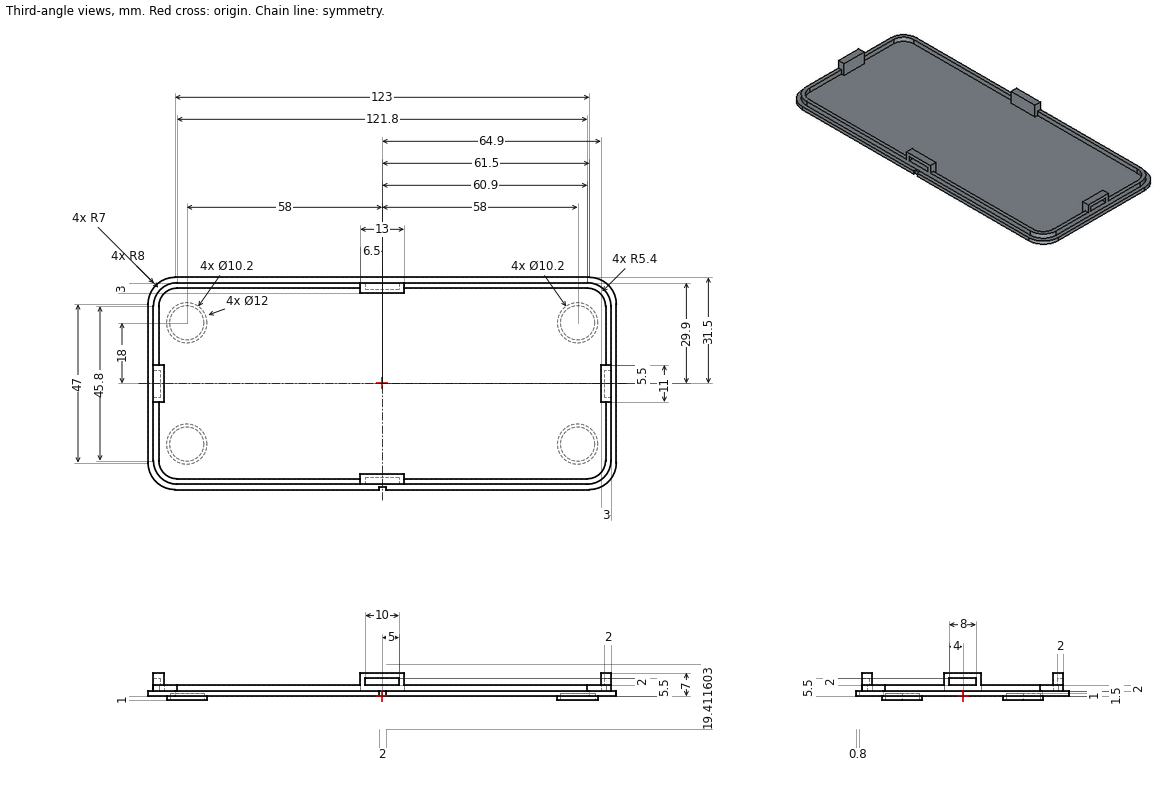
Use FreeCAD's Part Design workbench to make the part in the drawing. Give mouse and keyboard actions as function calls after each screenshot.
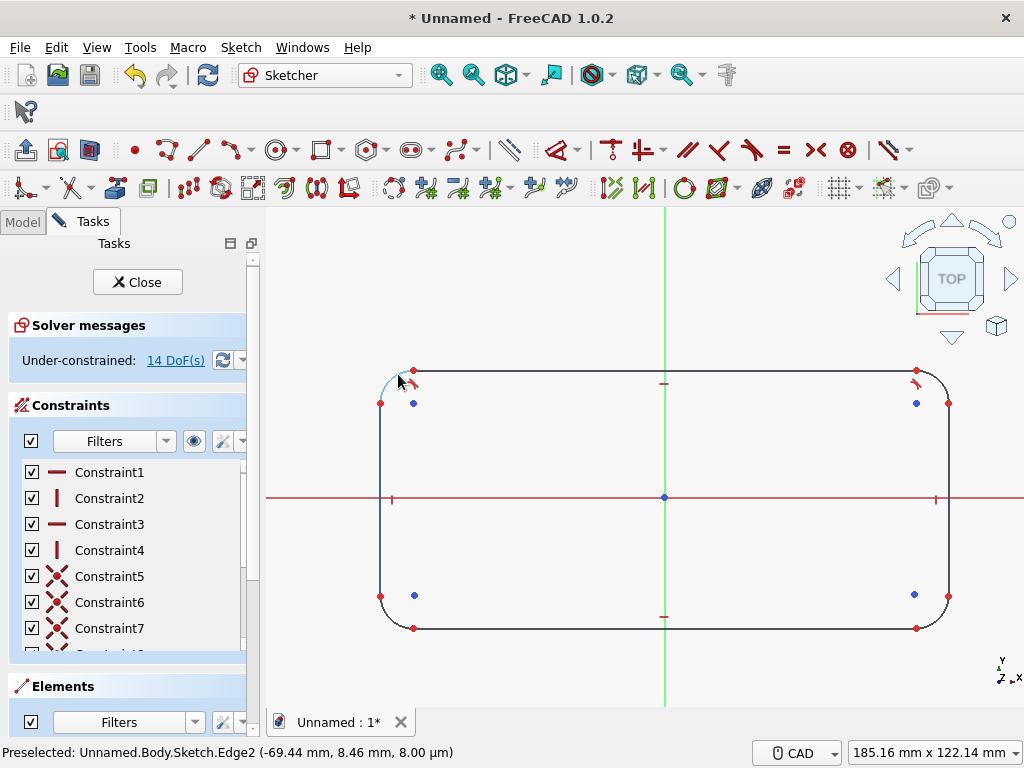
click(398, 374)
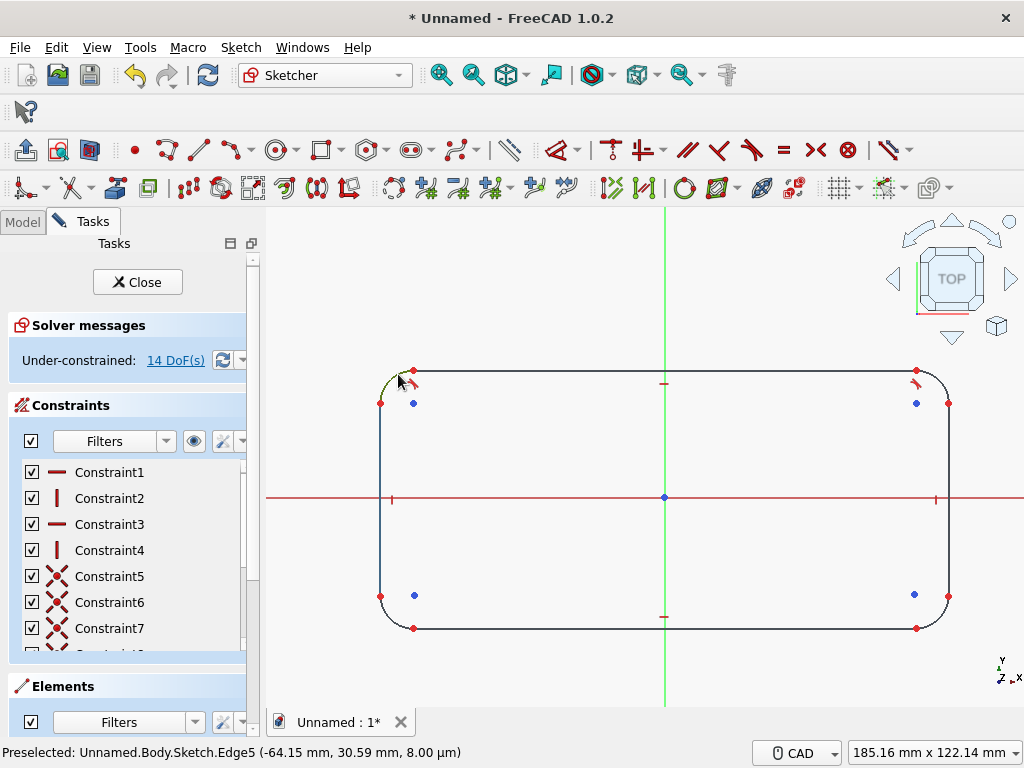
key(t)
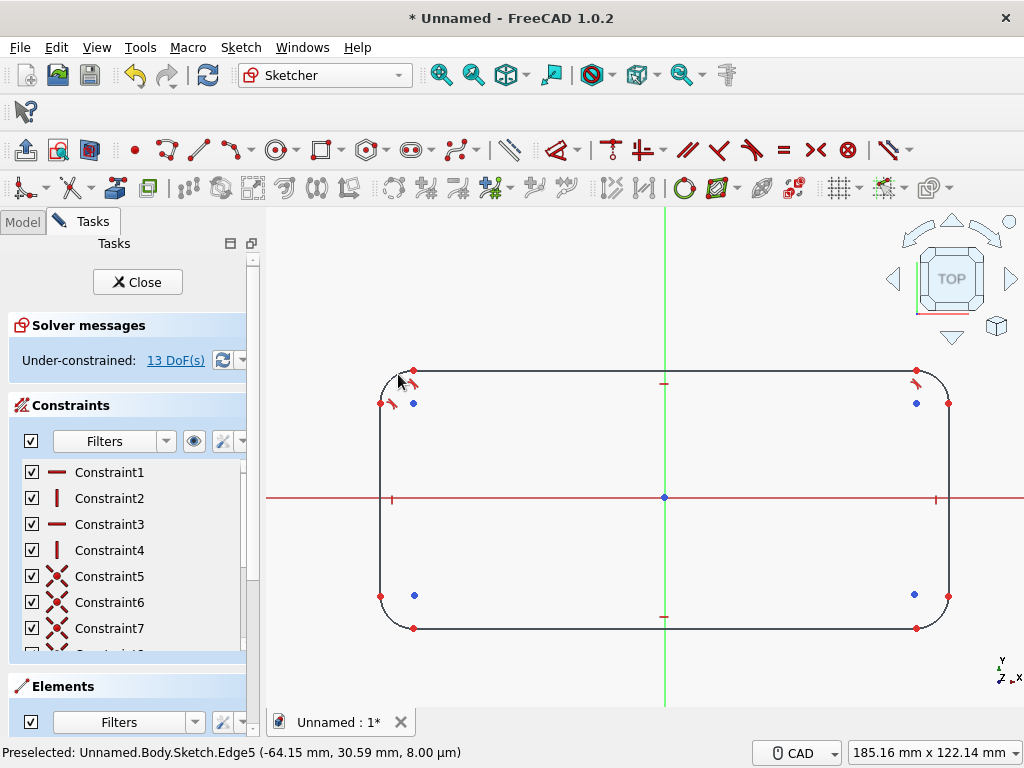
click(380, 461)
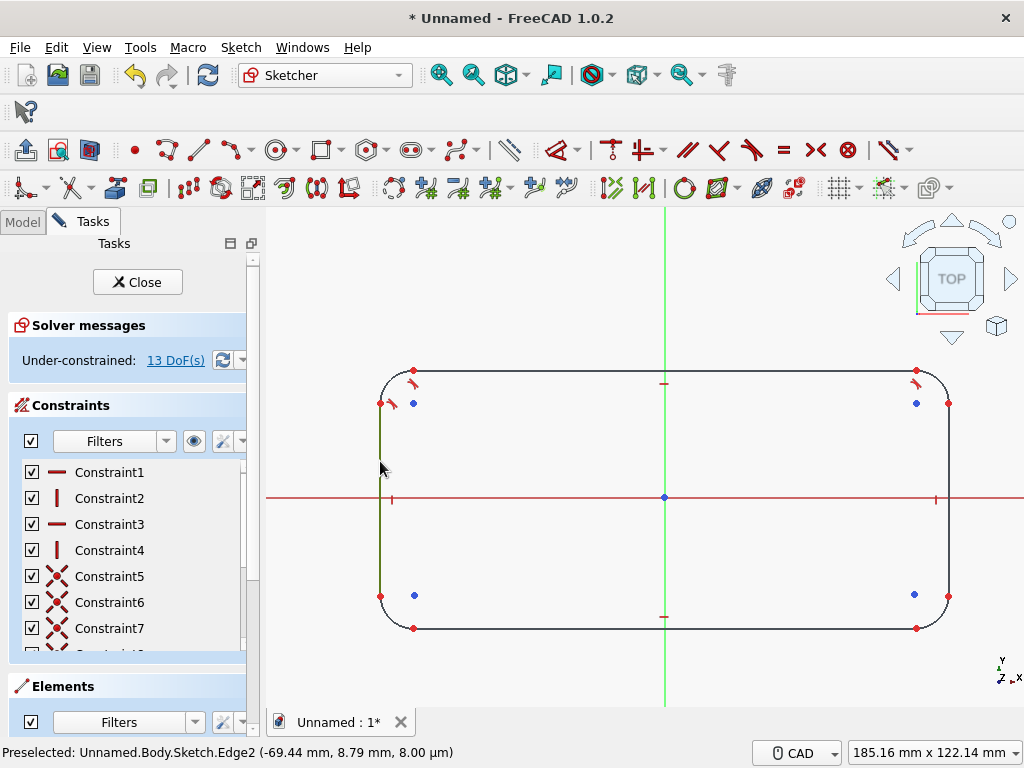
click(384, 611)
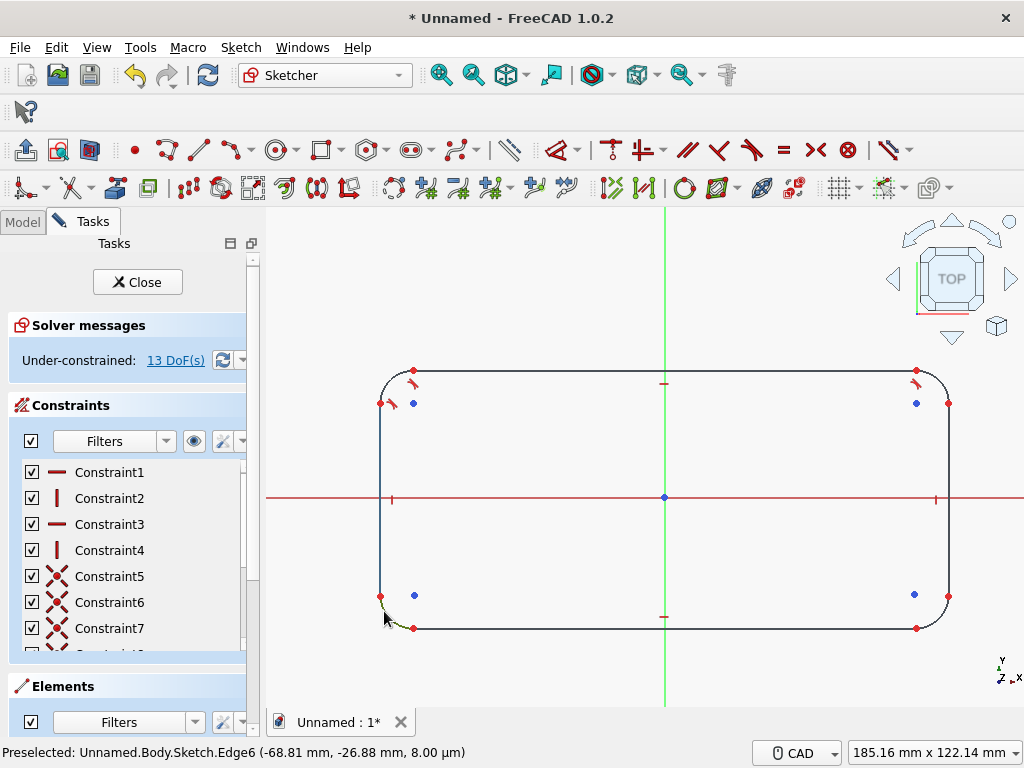
key(t)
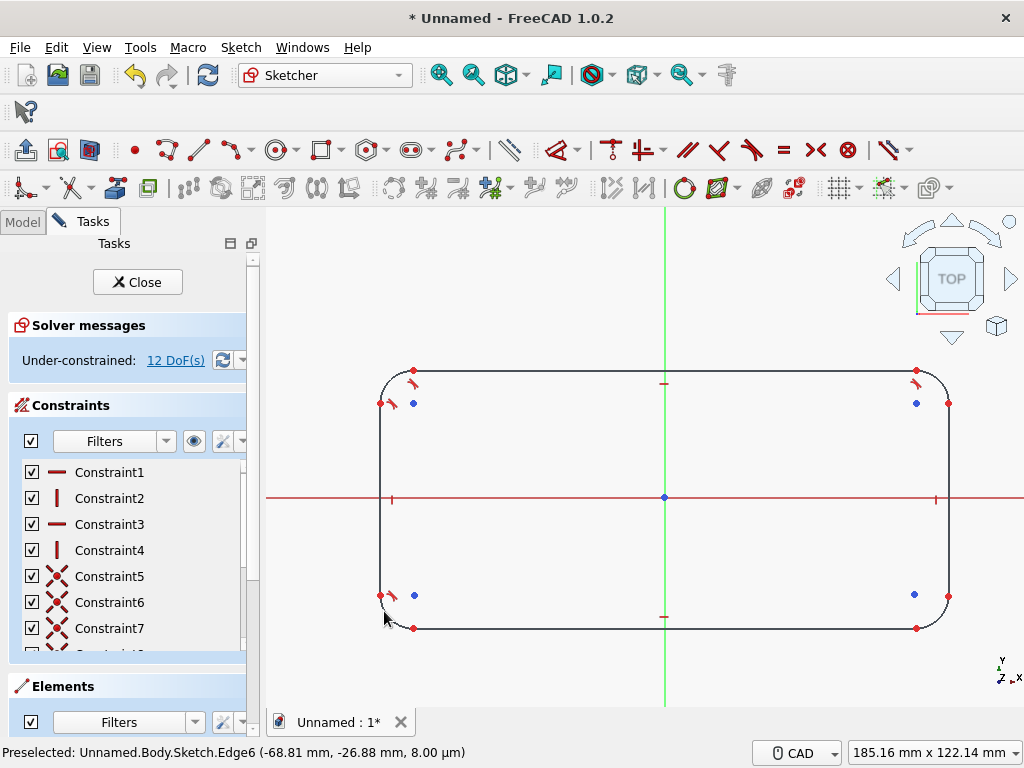
click(564, 629)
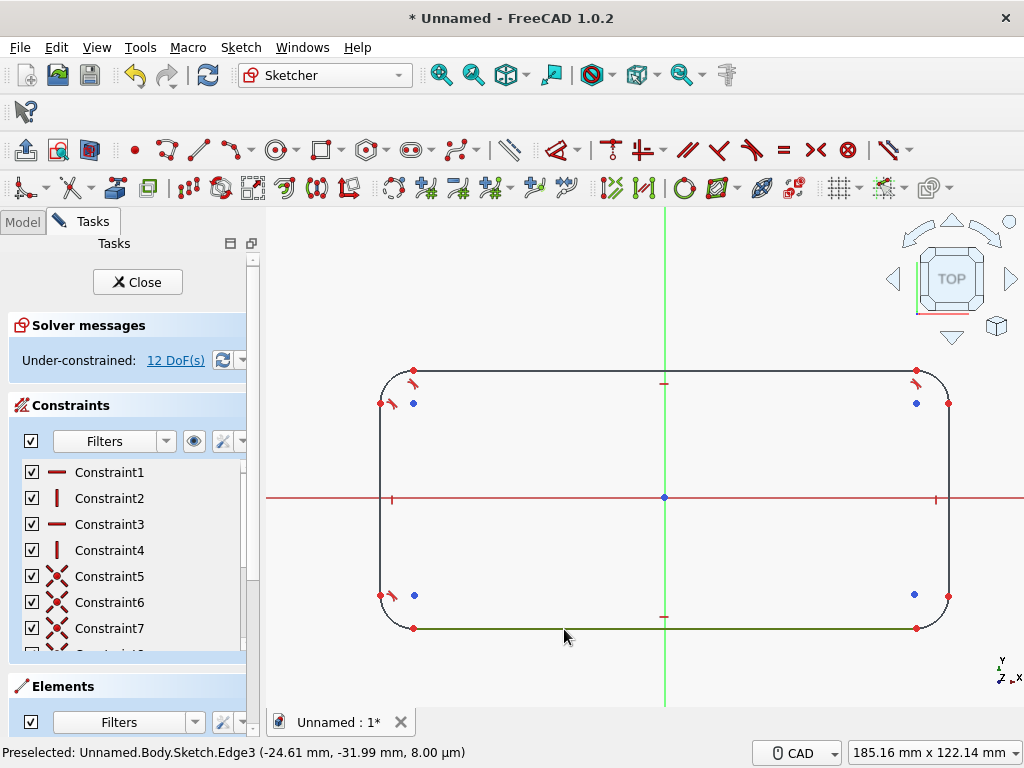
click(384, 610)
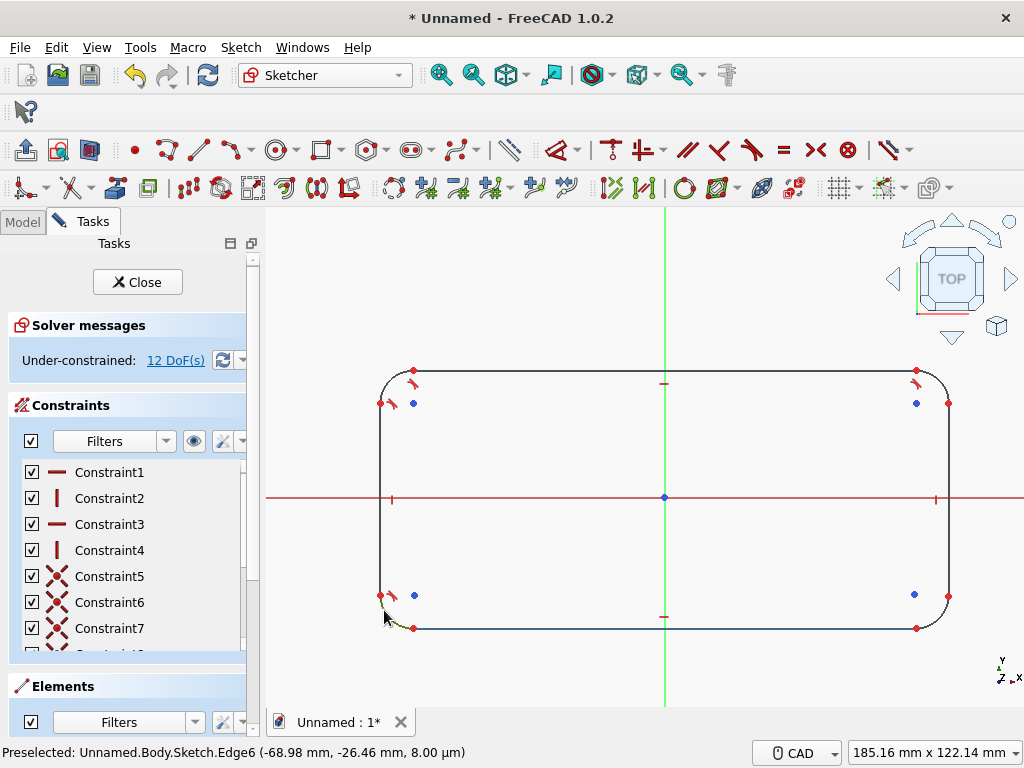
key(t)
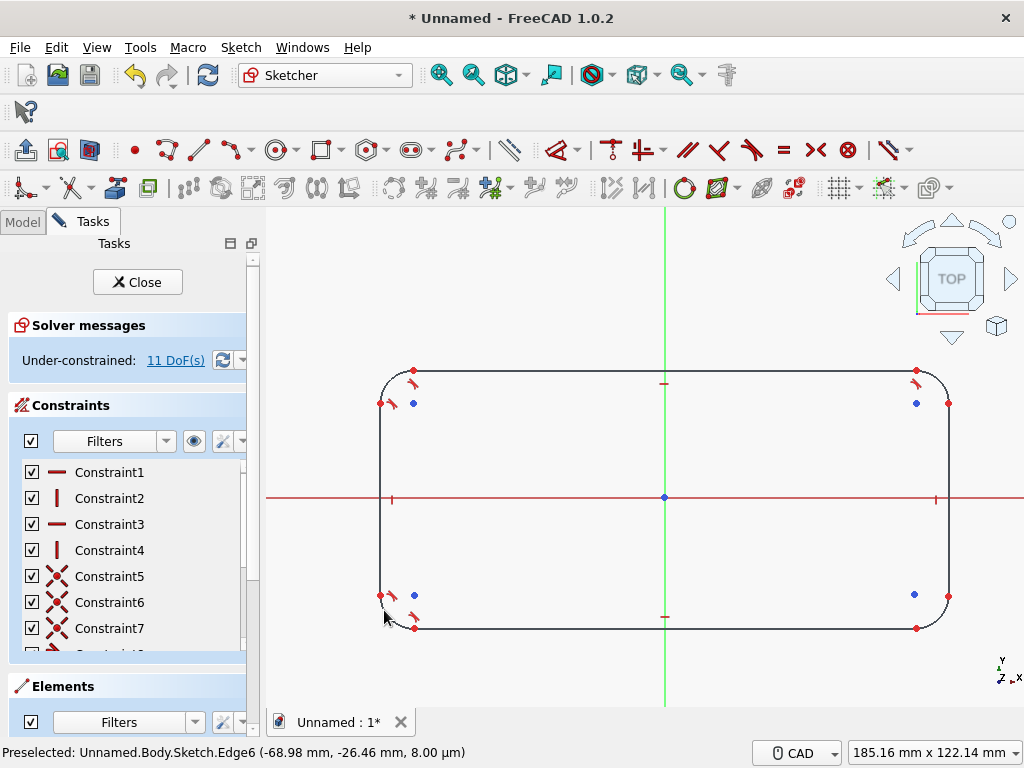
click(565, 629)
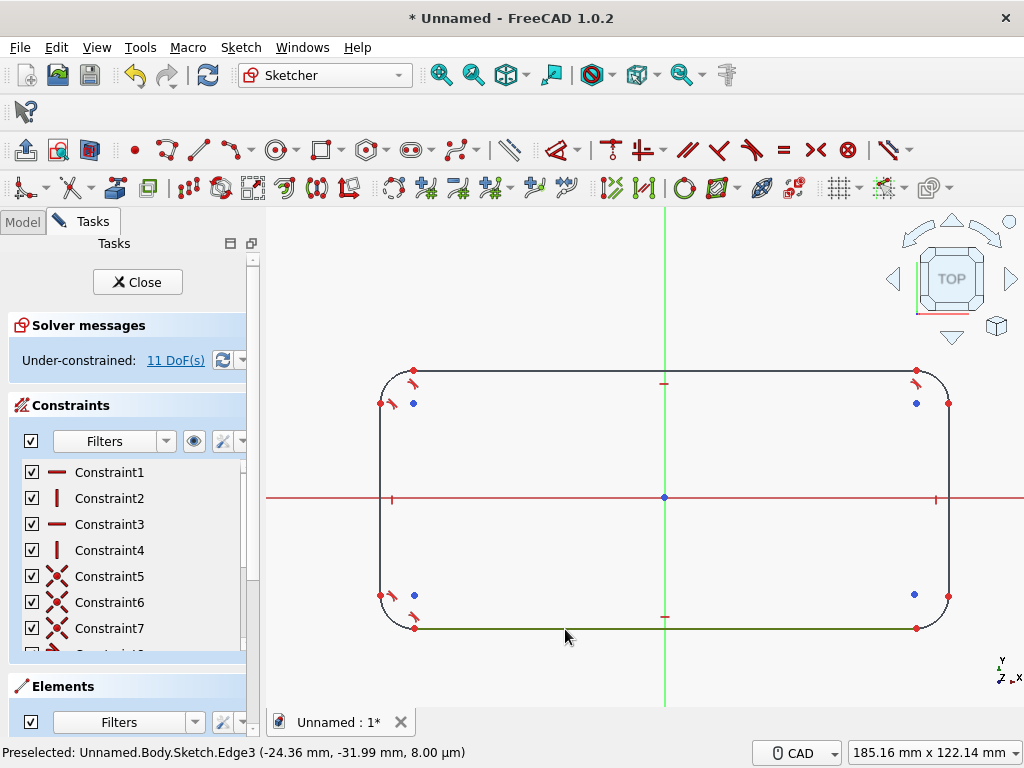
scroll(397, 374, down, 2)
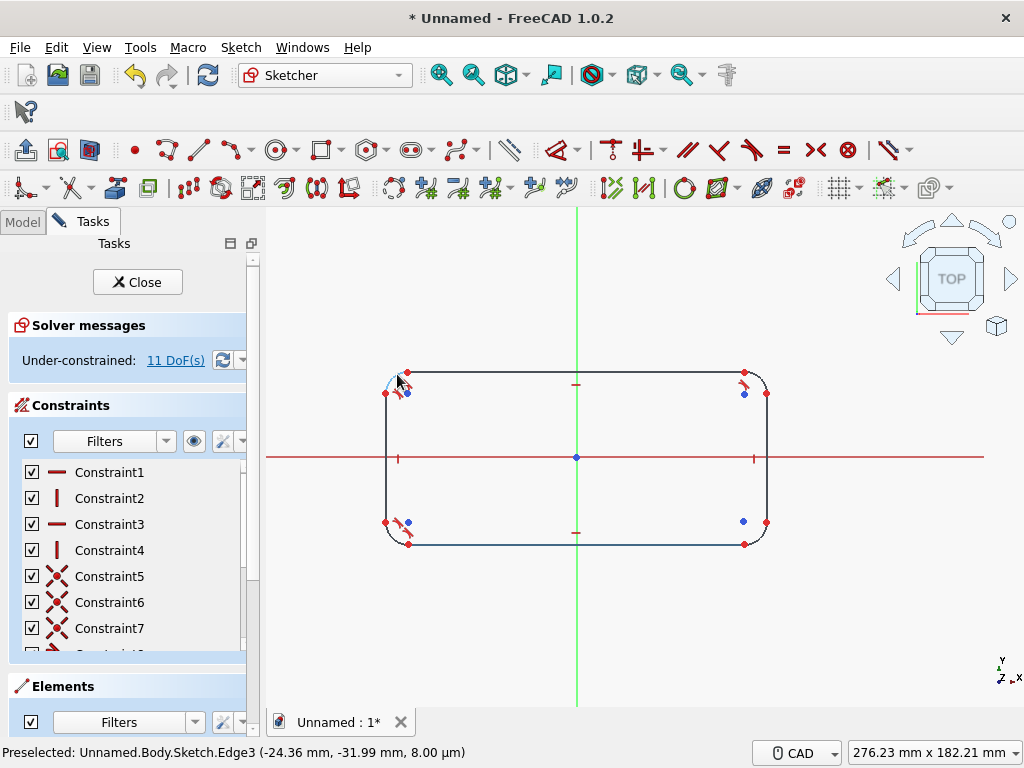
scroll(755, 542, up, 2)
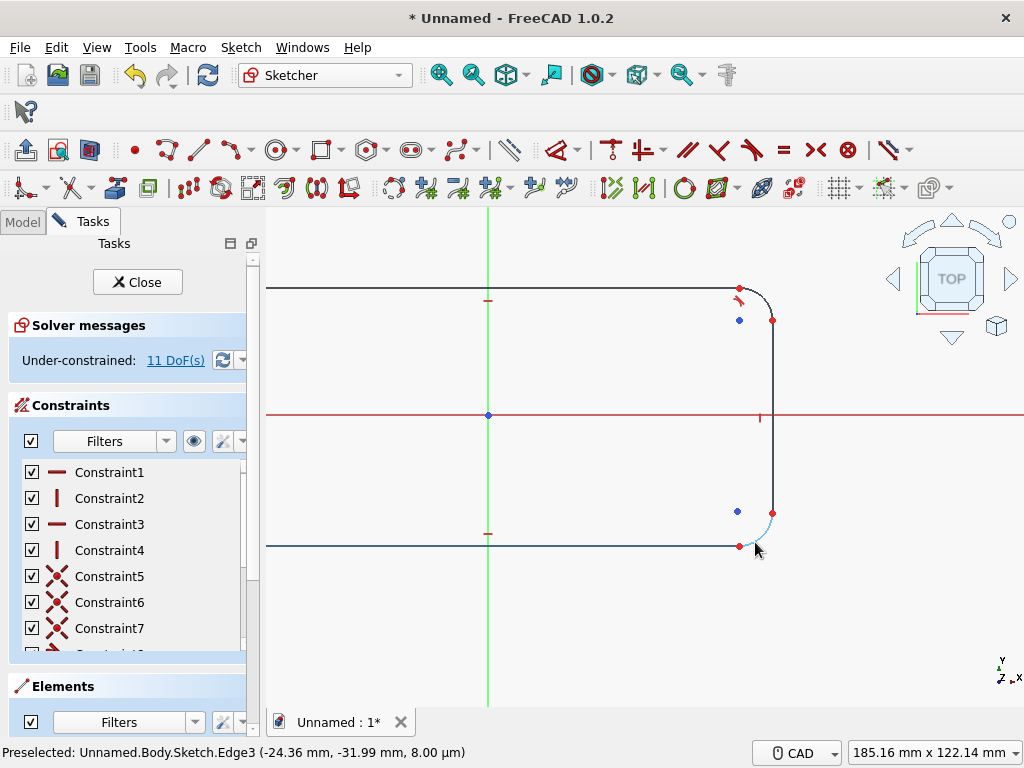
click(754, 542)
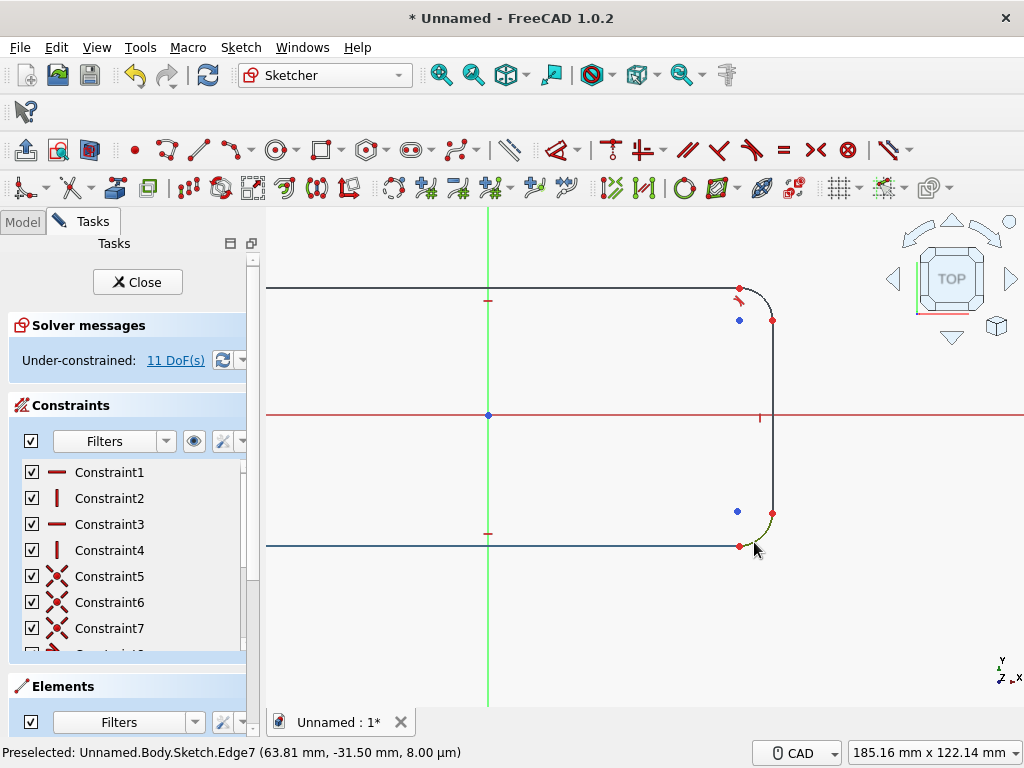
key(t)